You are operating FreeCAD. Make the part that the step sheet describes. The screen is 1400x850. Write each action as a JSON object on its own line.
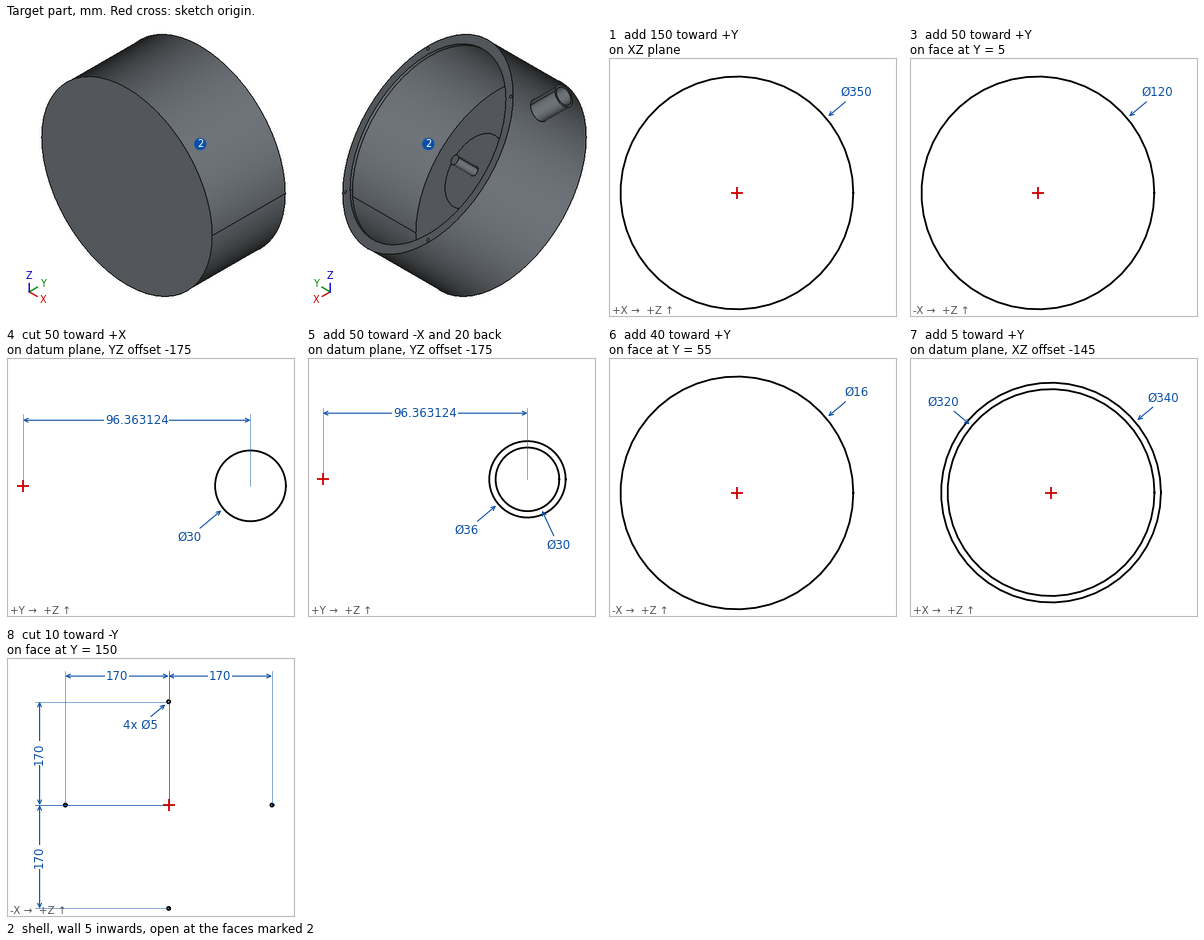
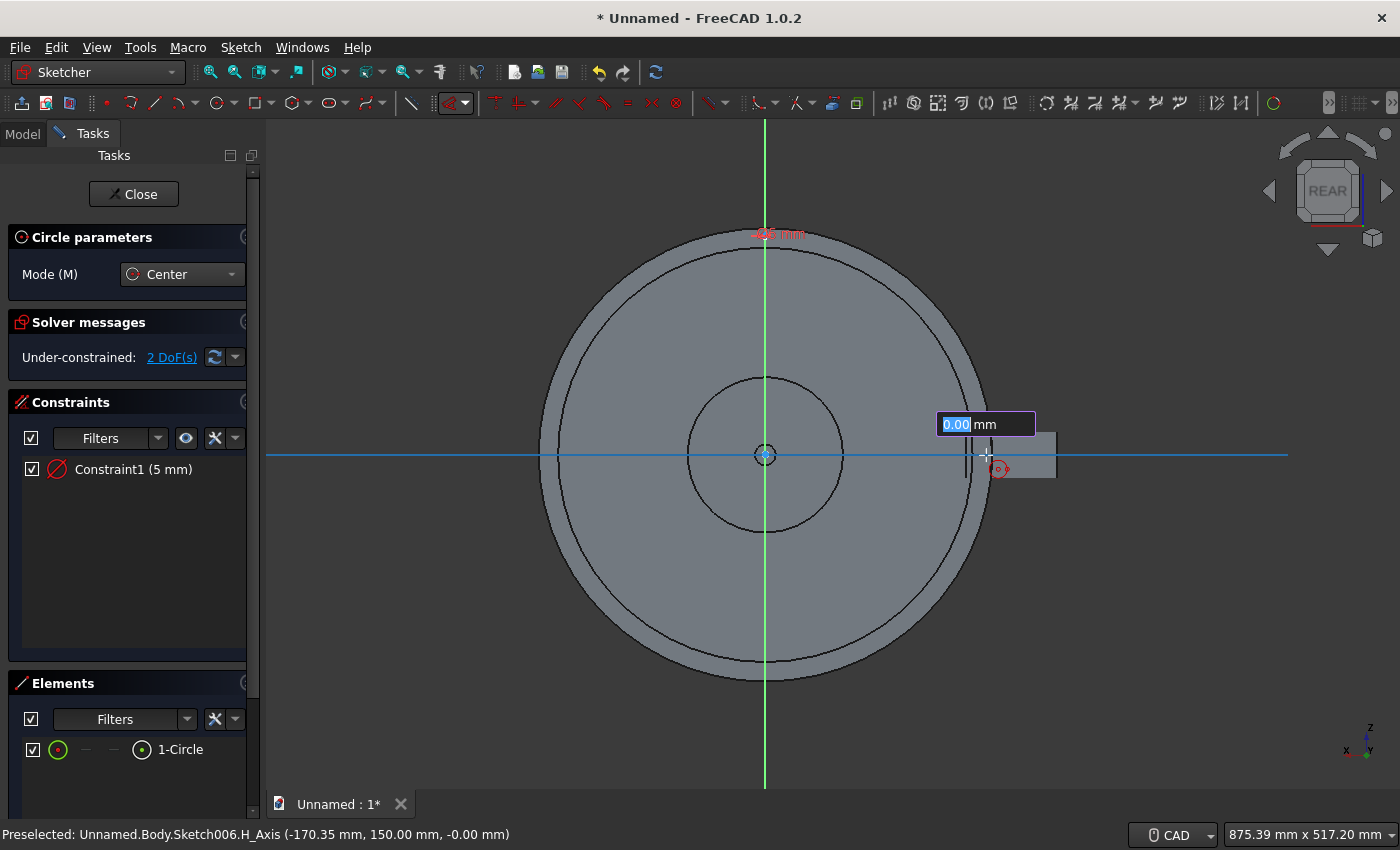
{"action": "scroll", "coordinate": [984, 458], "scroll_direction": "up", "scroll_amount": 9}
{"action": "mouse_move", "coordinate": [983, 455]}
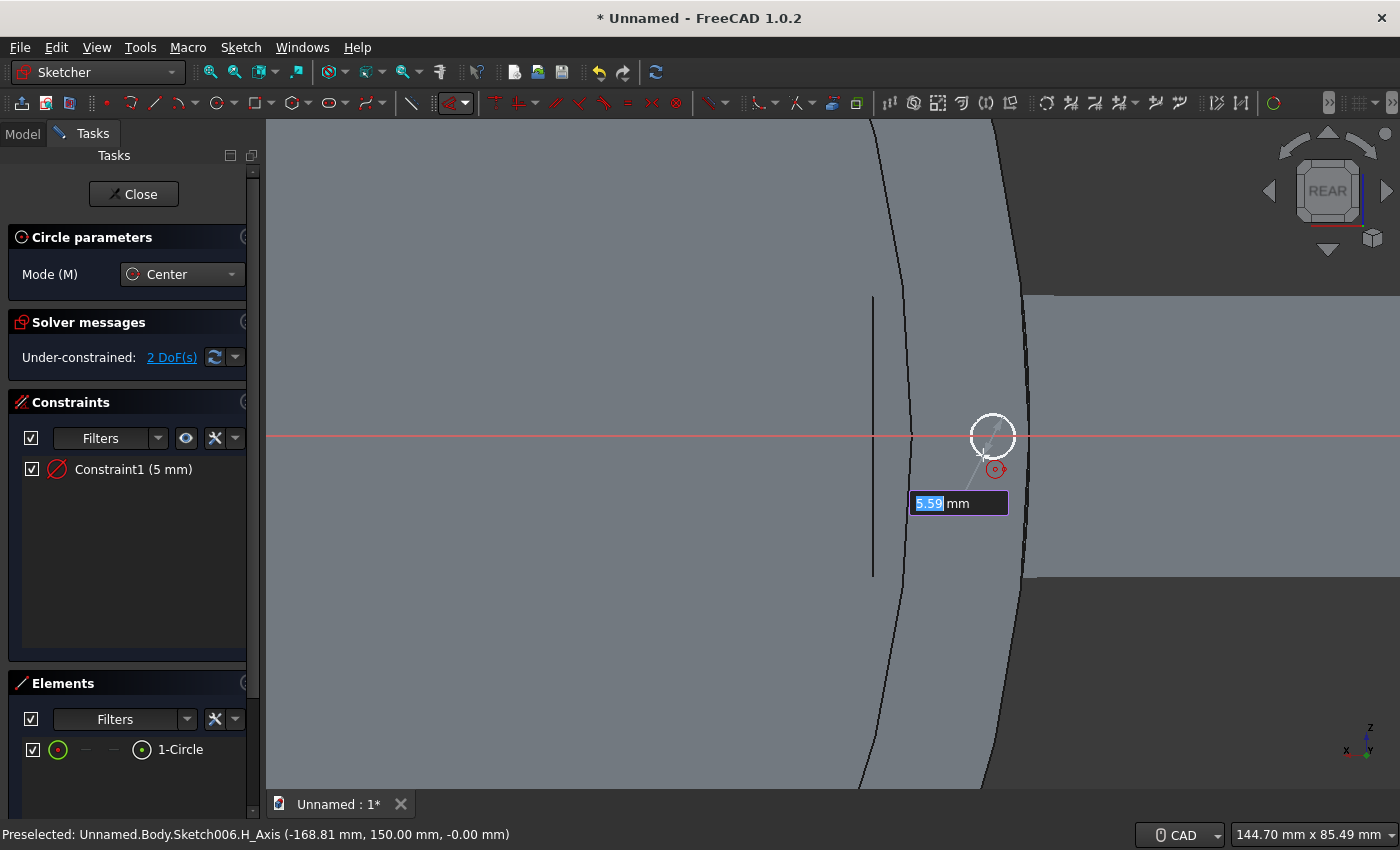
{"action": "type", "text": "5"}
{"action": "key", "text": "Return"}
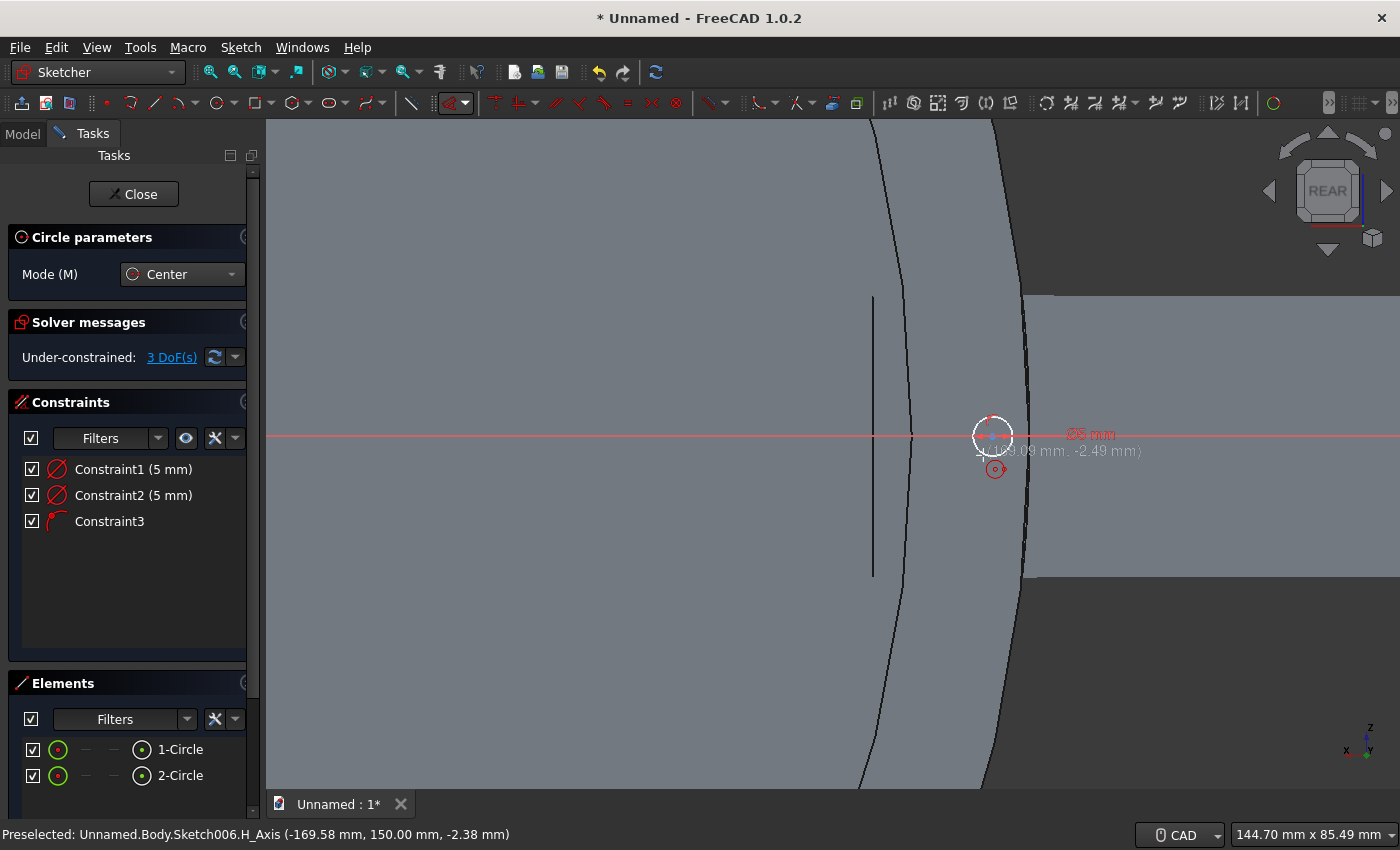
{"action": "scroll", "coordinate": [984, 457], "scroll_direction": "down", "scroll_amount": 9}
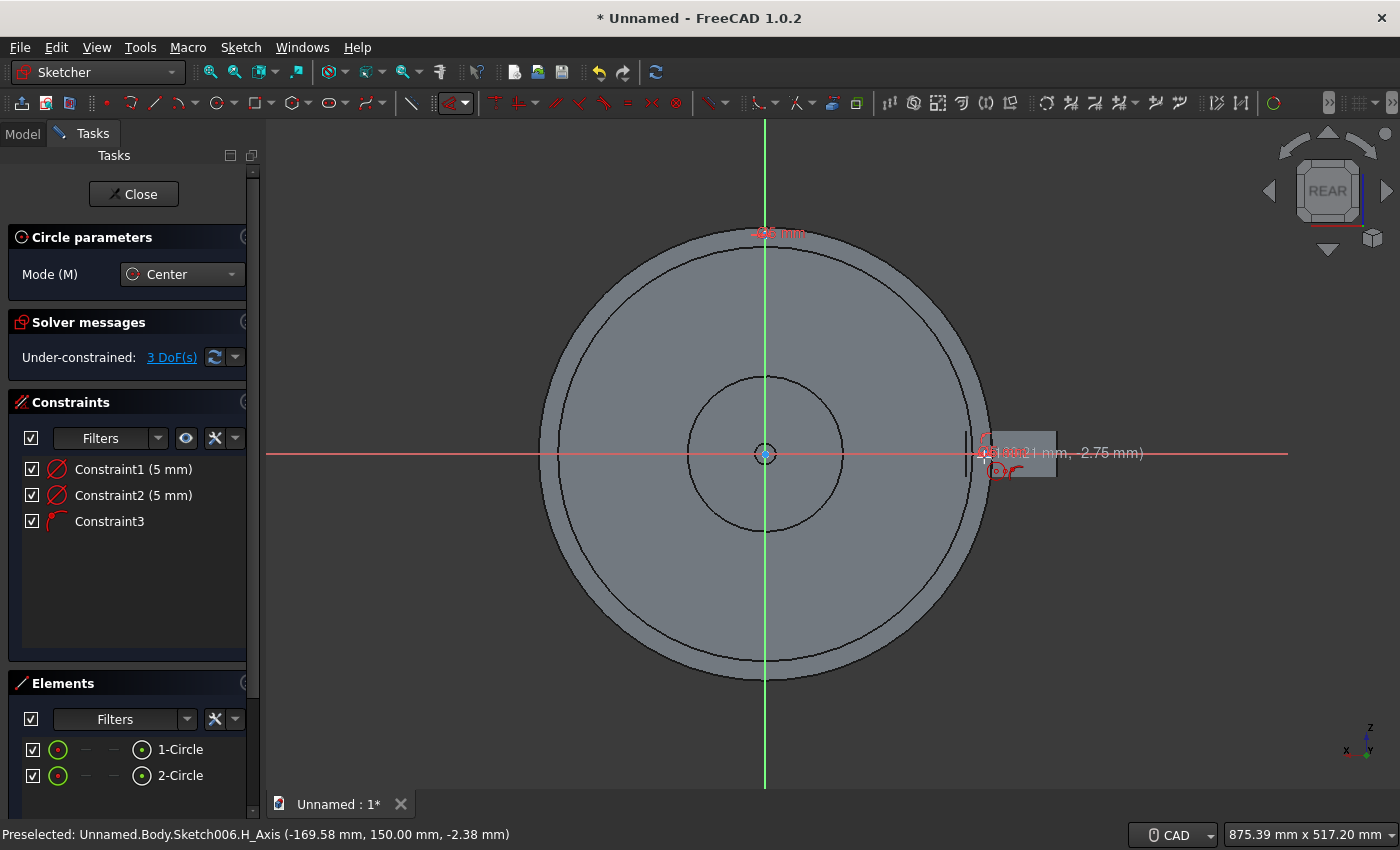
{"action": "scroll", "coordinate": [765, 674], "scroll_direction": "up", "scroll_amount": 10}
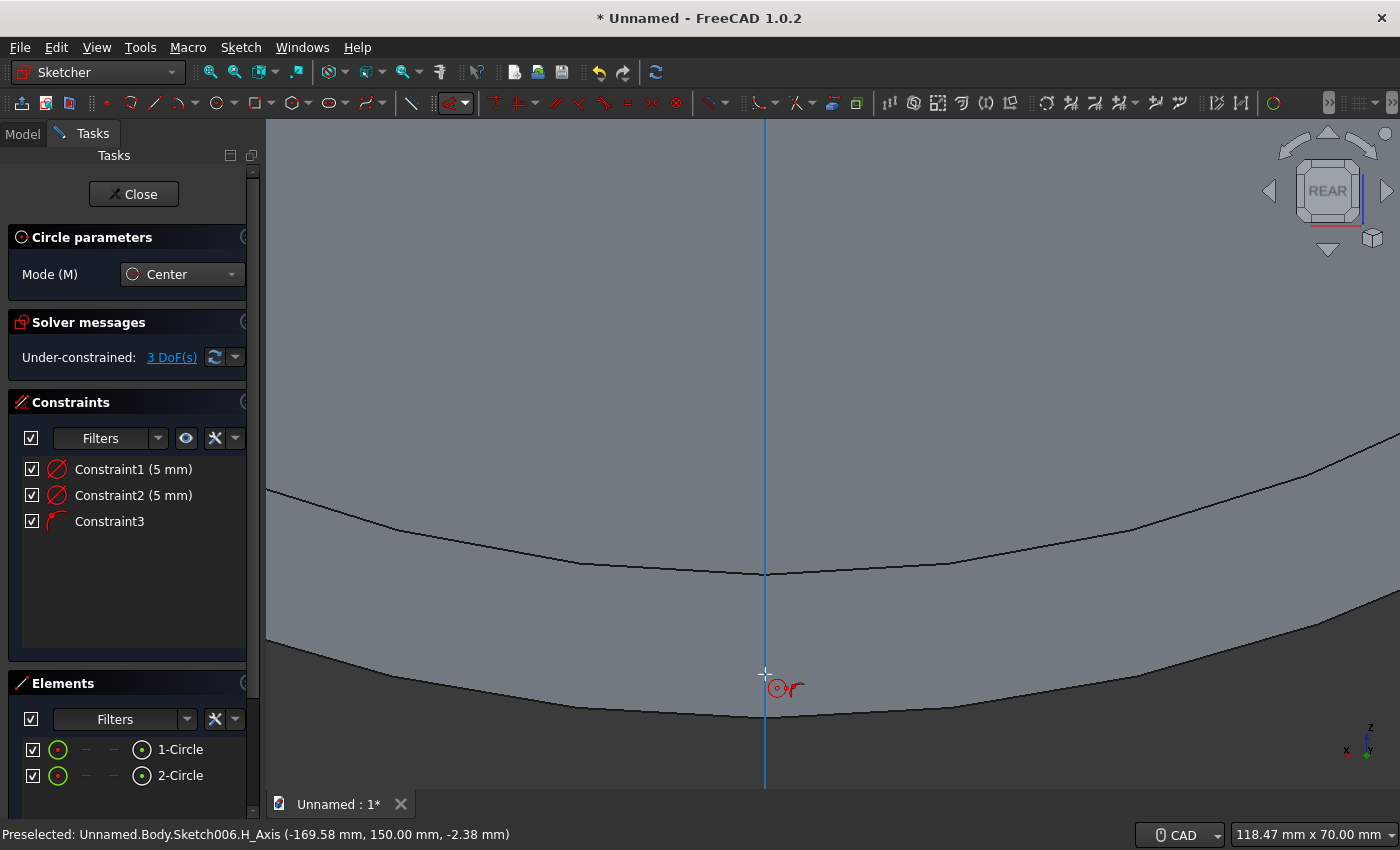
{"action": "scroll", "coordinate": [764, 675], "scroll_direction": "down", "scroll_amount": 10}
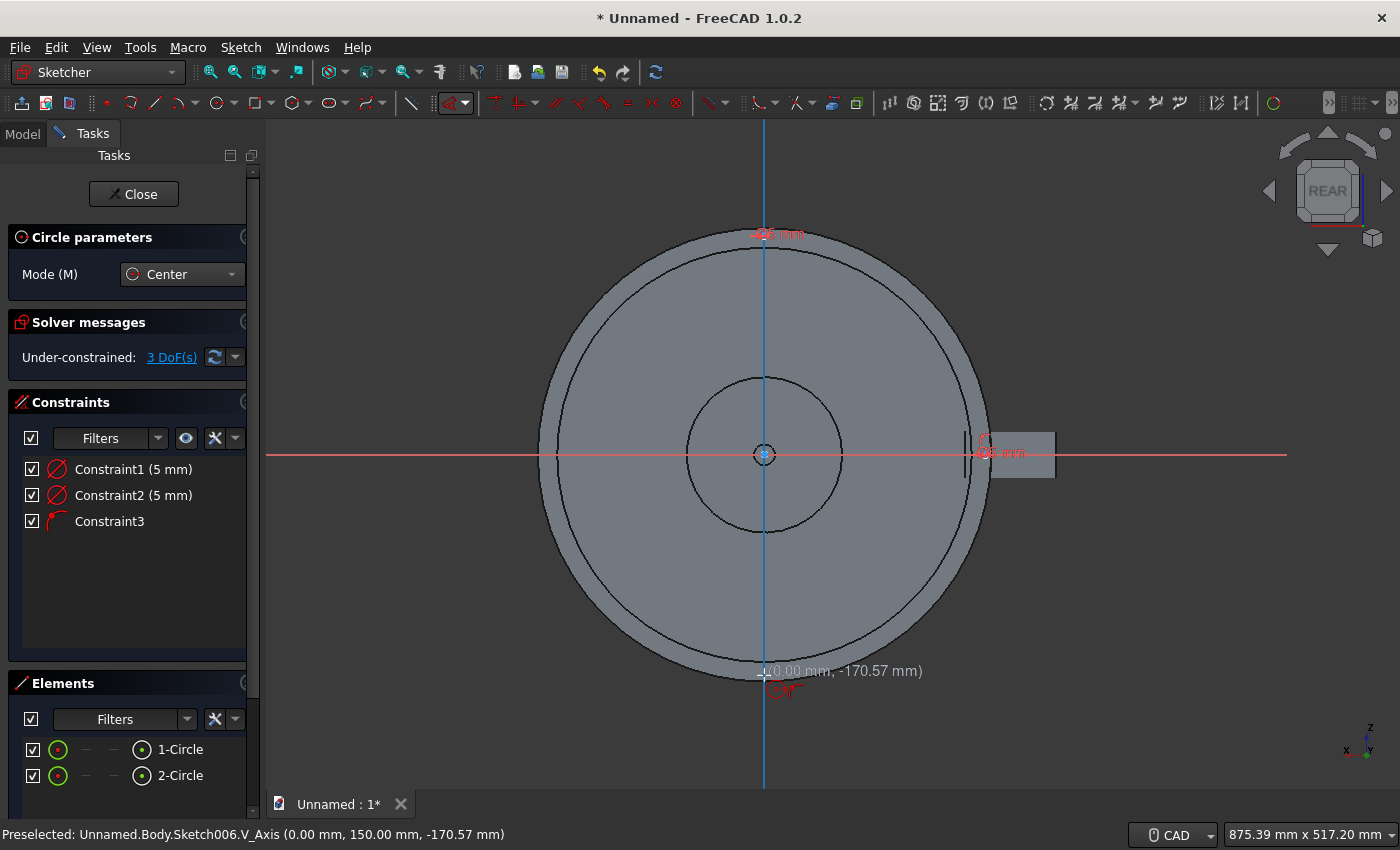
{"action": "left_click", "coordinate": [764, 675]}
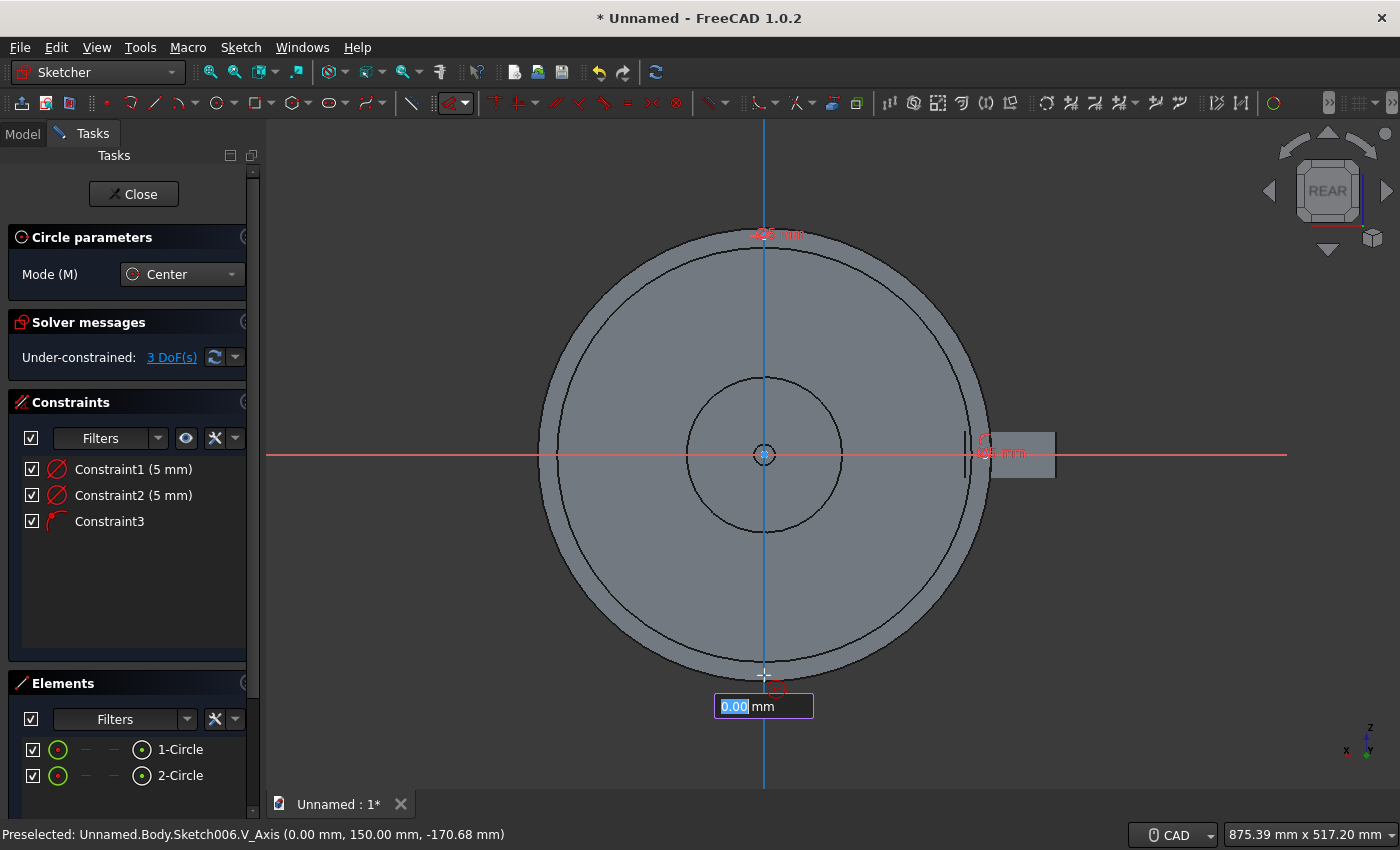
{"action": "scroll", "coordinate": [768, 674], "scroll_direction": "up", "scroll_amount": 9}
{"action": "mouse_move", "coordinate": [763, 670]}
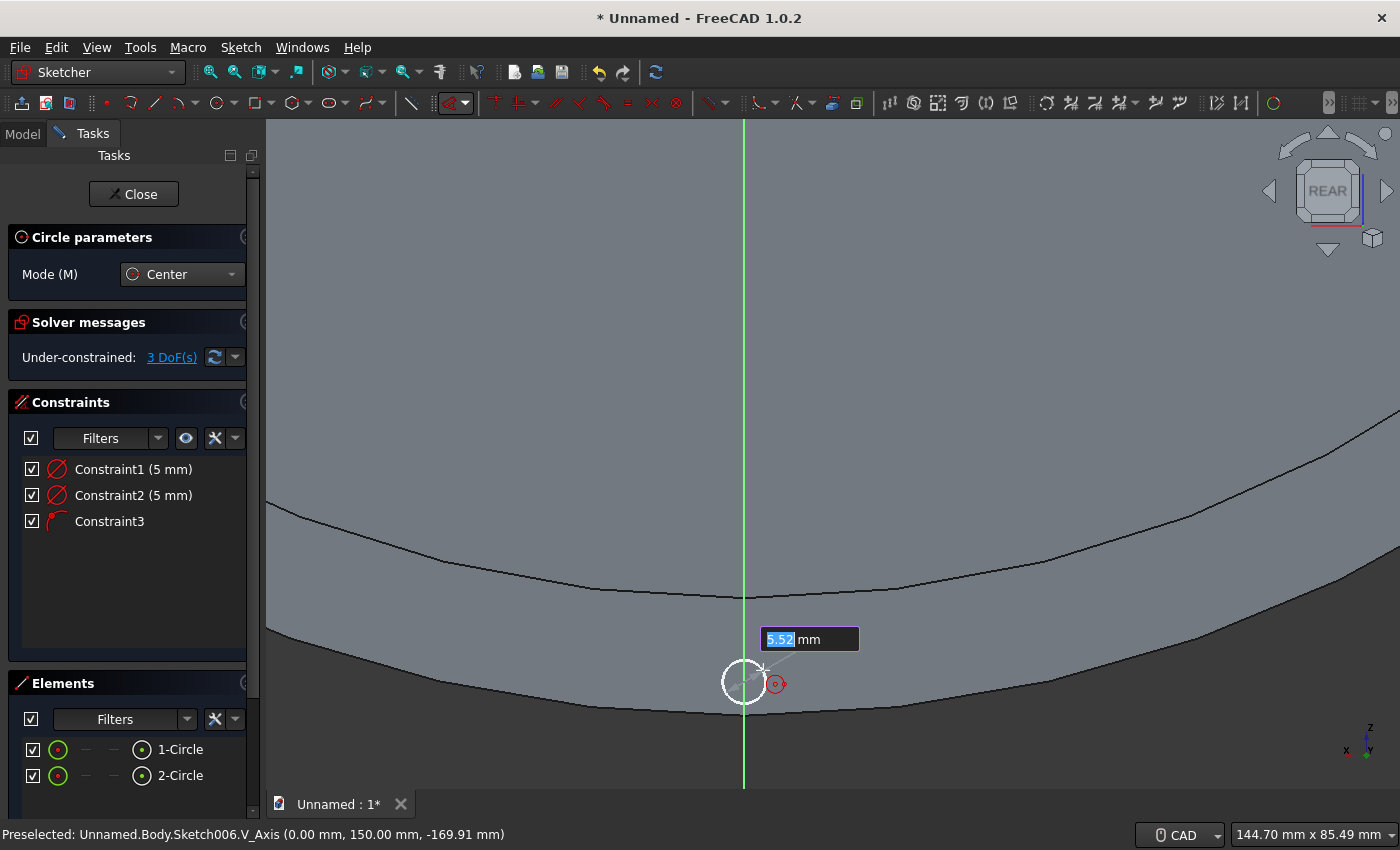
{"action": "type", "text": "5"}
{"action": "key", "text": "Return"}